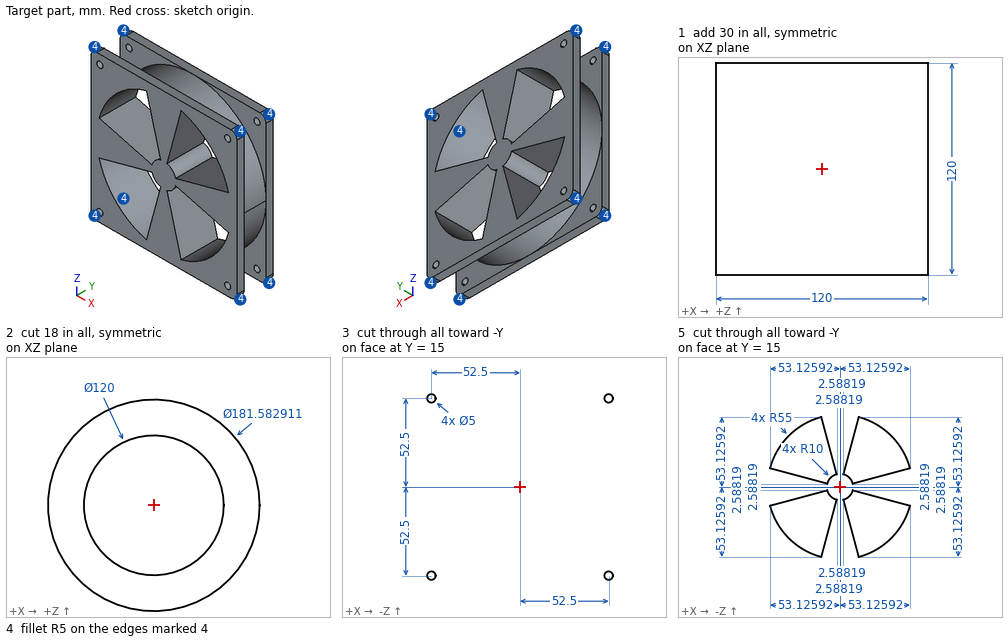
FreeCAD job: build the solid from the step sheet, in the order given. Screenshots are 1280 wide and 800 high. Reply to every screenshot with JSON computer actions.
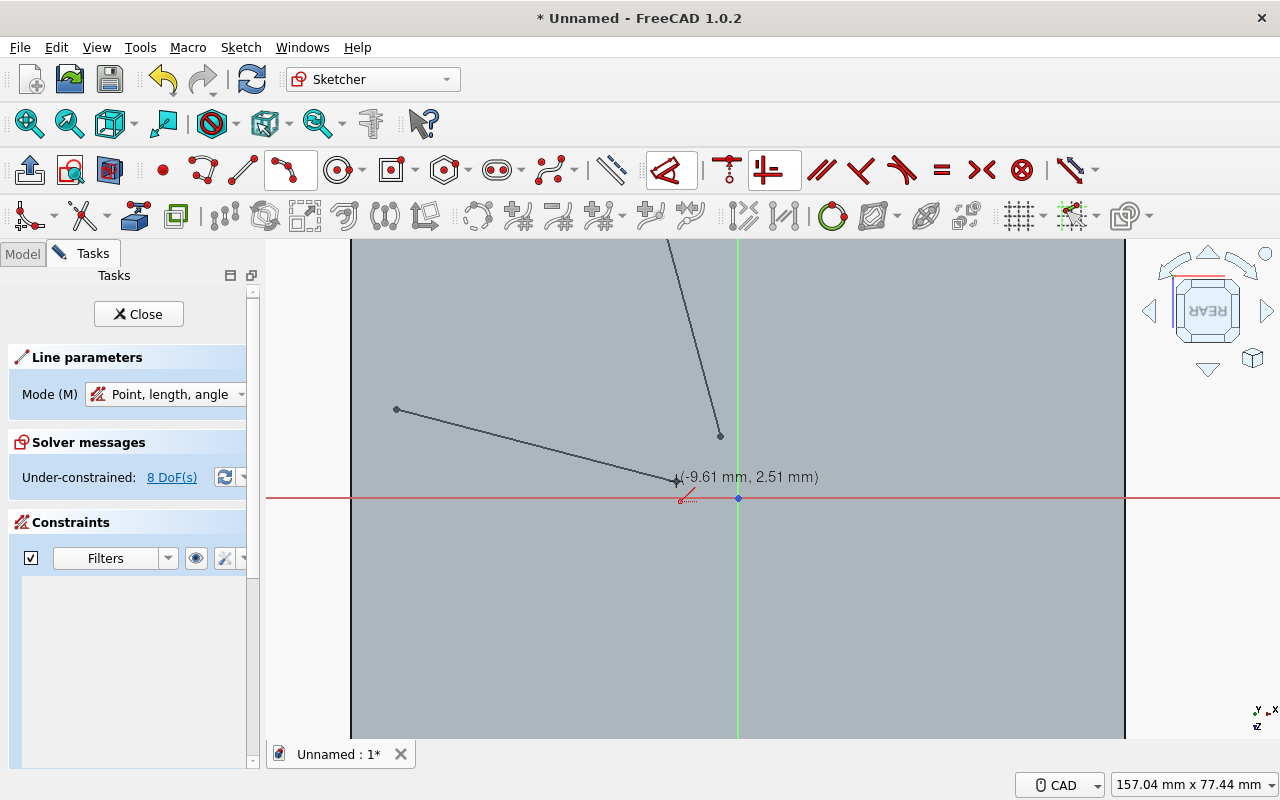
{"action": "left_click", "coordinate": [284, 170]}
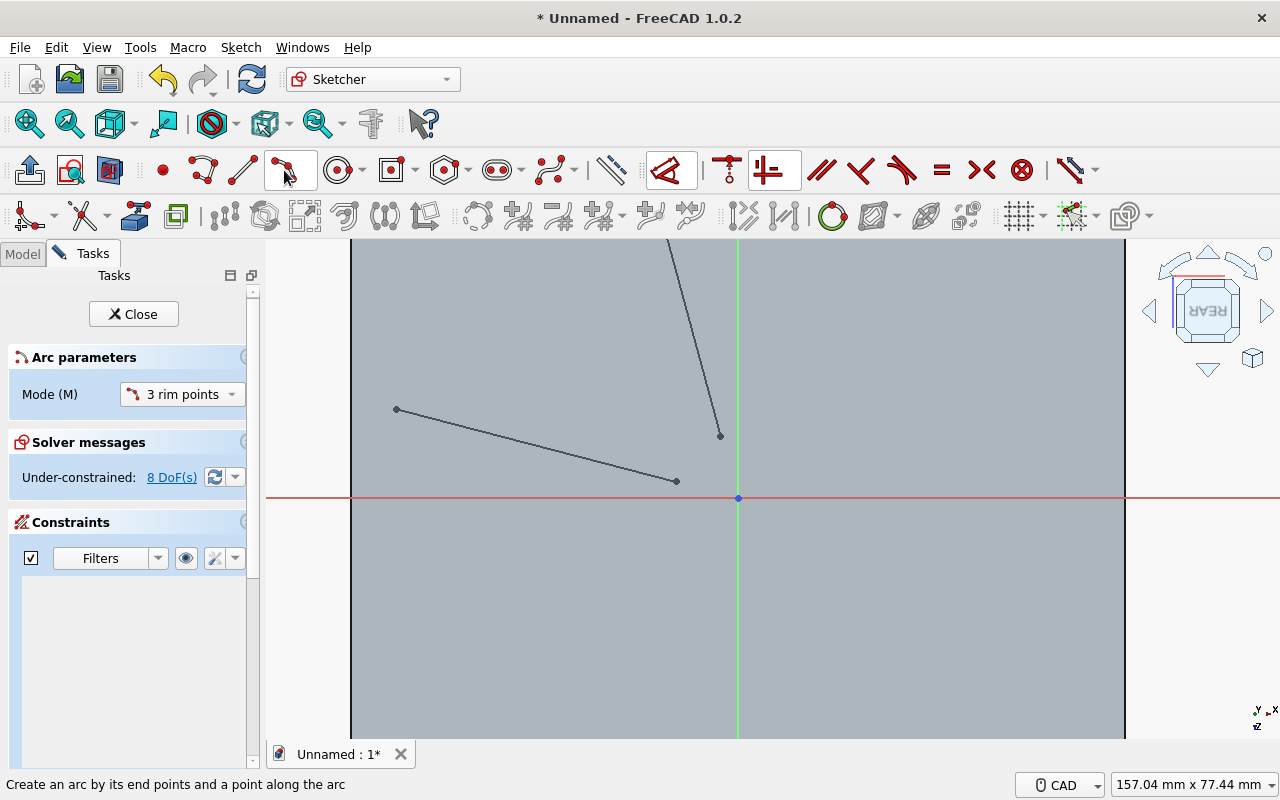
{"action": "scroll", "coordinate": [677, 481], "scroll_direction": "down", "scroll_amount": 4}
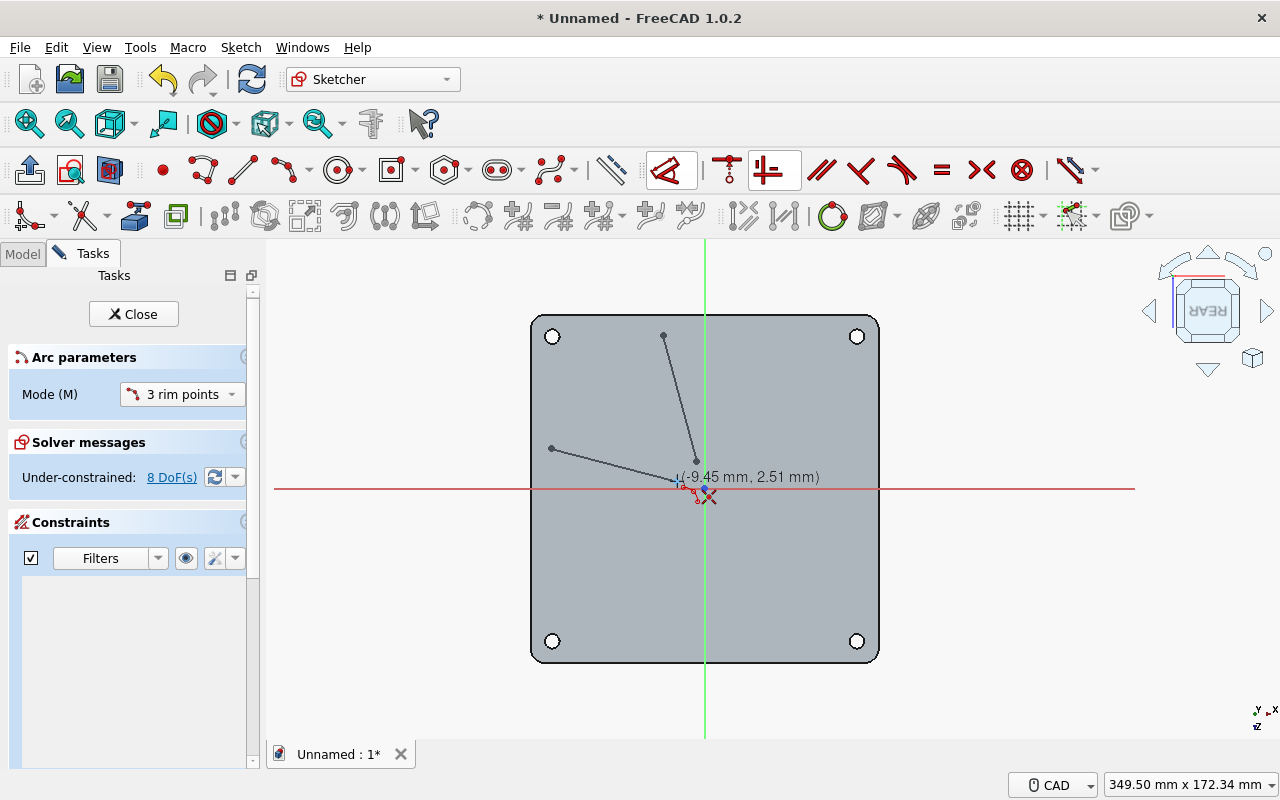
{"action": "left_click", "coordinate": [663, 336]}
{"action": "left_click", "coordinate": [551, 449]}
{"action": "left_click", "coordinate": [592, 376]}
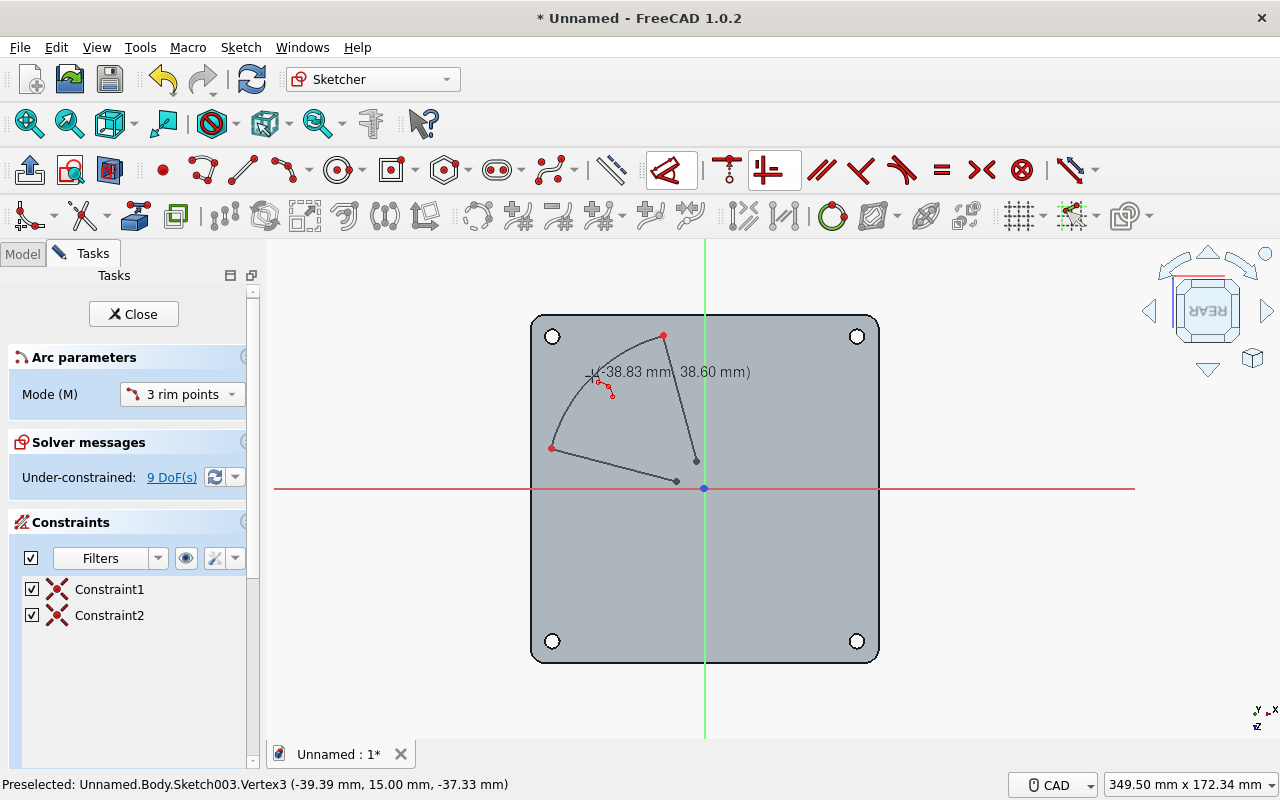
{"action": "scroll", "coordinate": [677, 481], "scroll_direction": "up", "scroll_amount": 4}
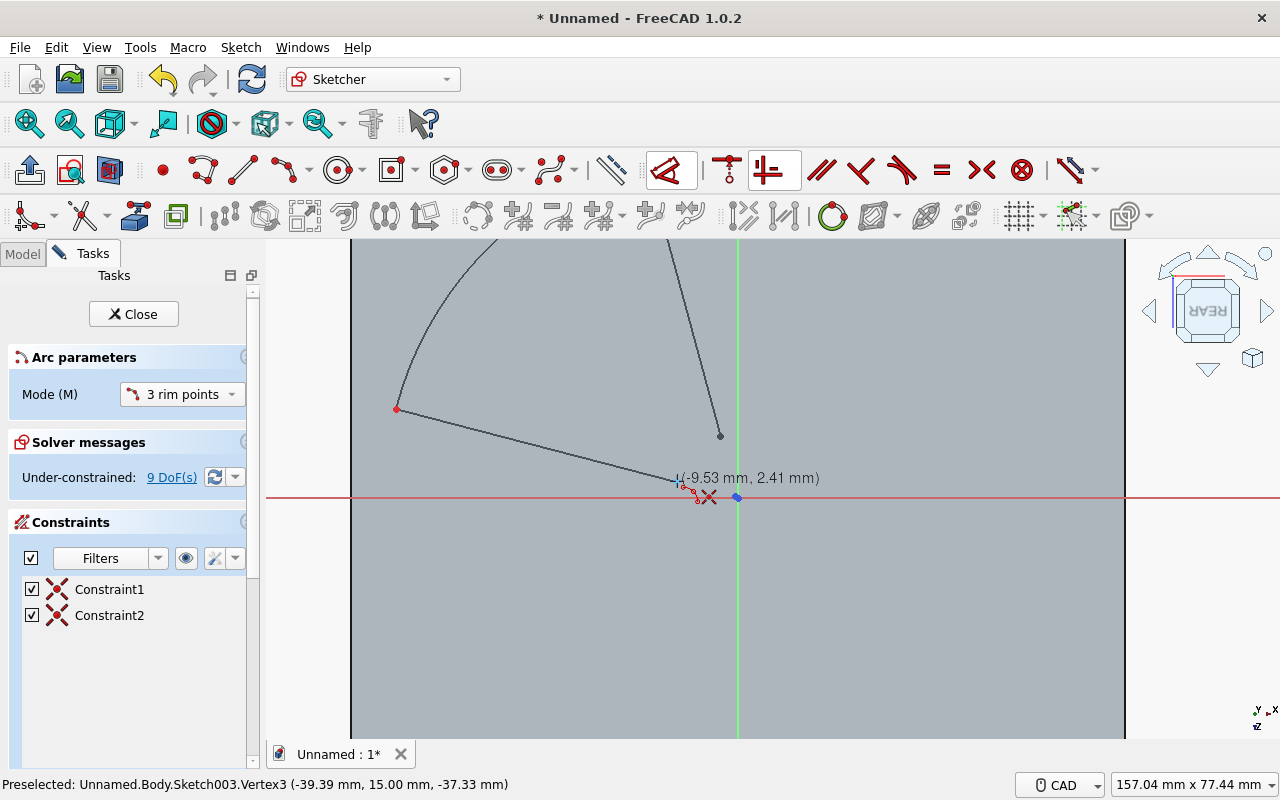
{"action": "left_click", "coordinate": [676, 482]}
{"action": "left_click", "coordinate": [721, 436]}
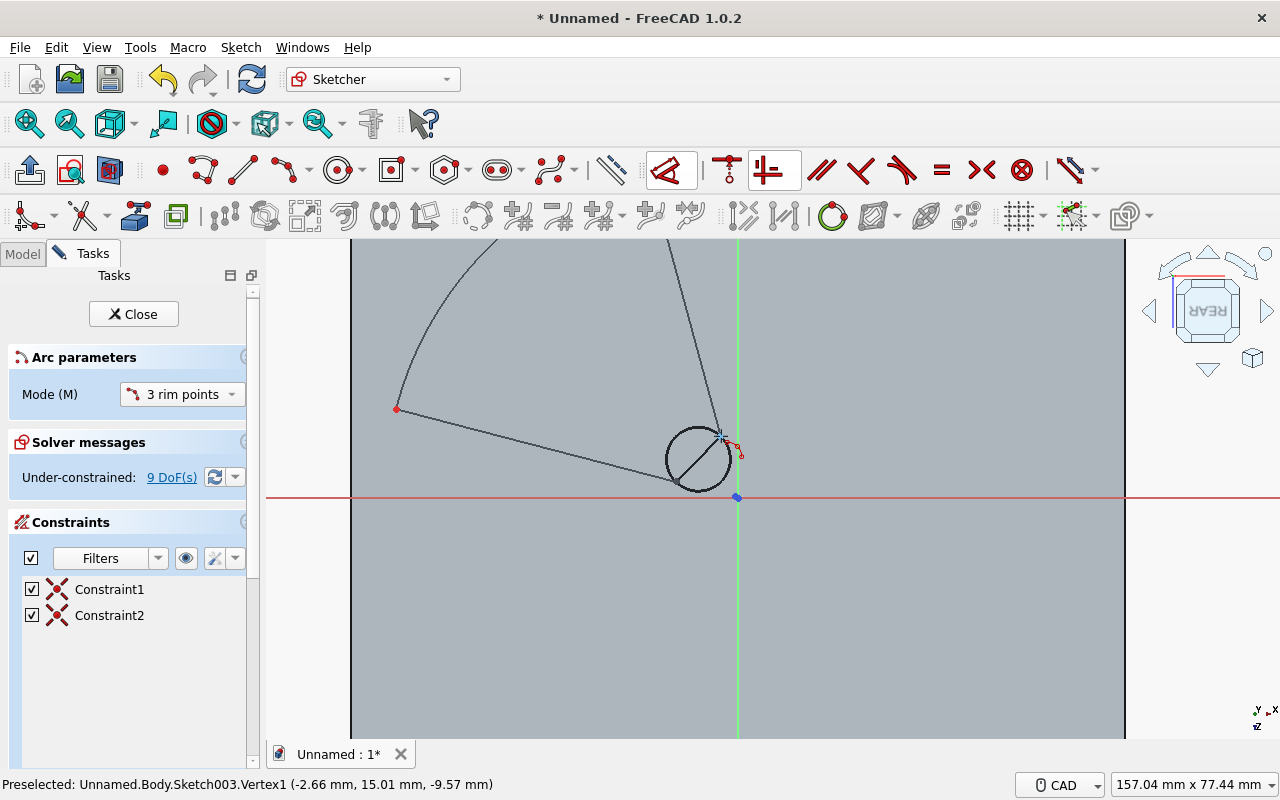
{"action": "scroll", "coordinate": [692, 453], "scroll_direction": "up", "scroll_amount": 4}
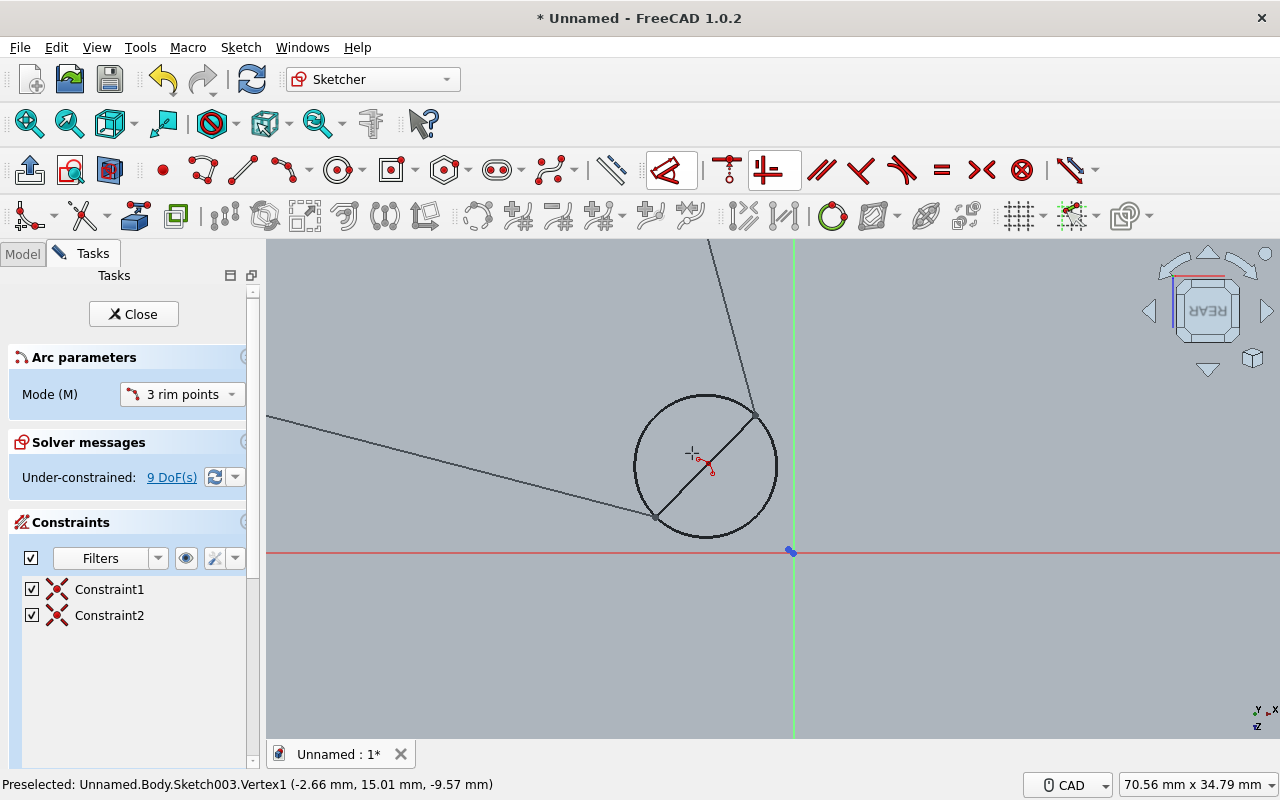
{"action": "left_click", "coordinate": [692, 451]}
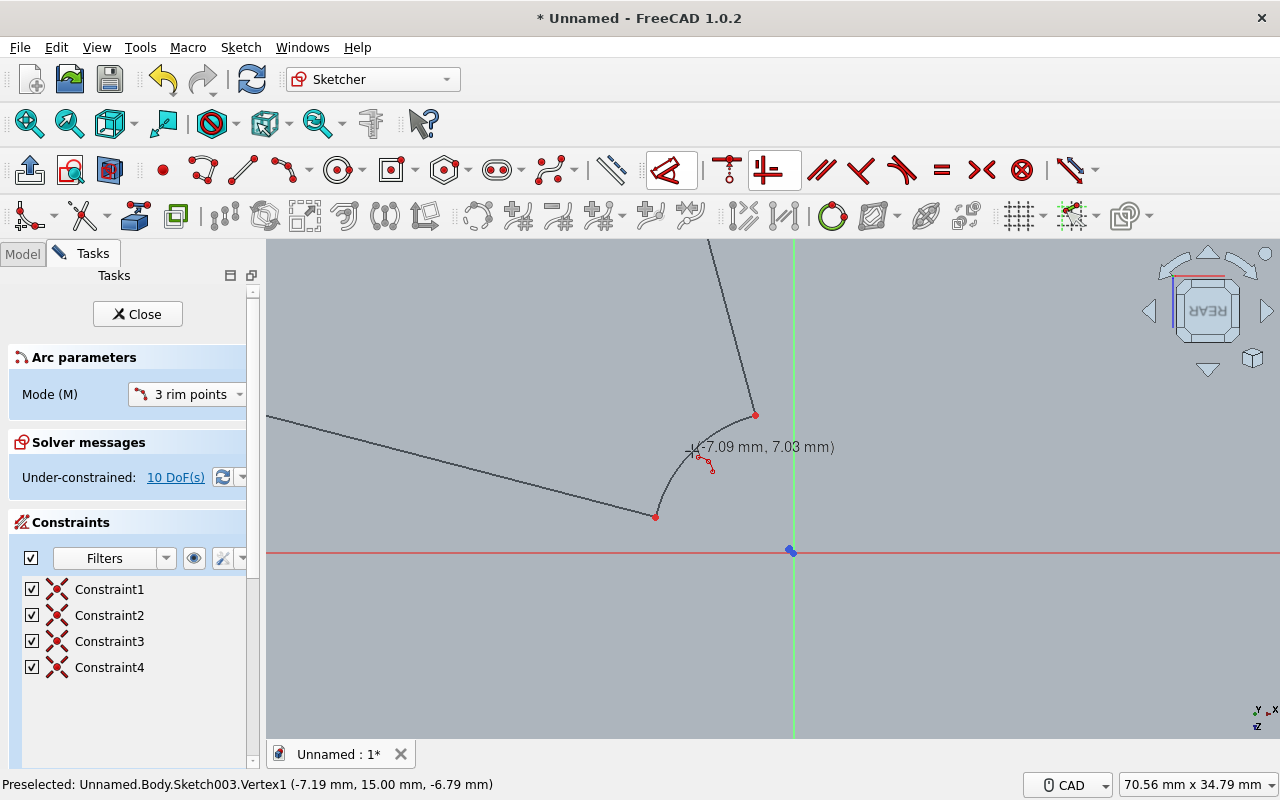
{"action": "left_click", "coordinate": [244, 170]}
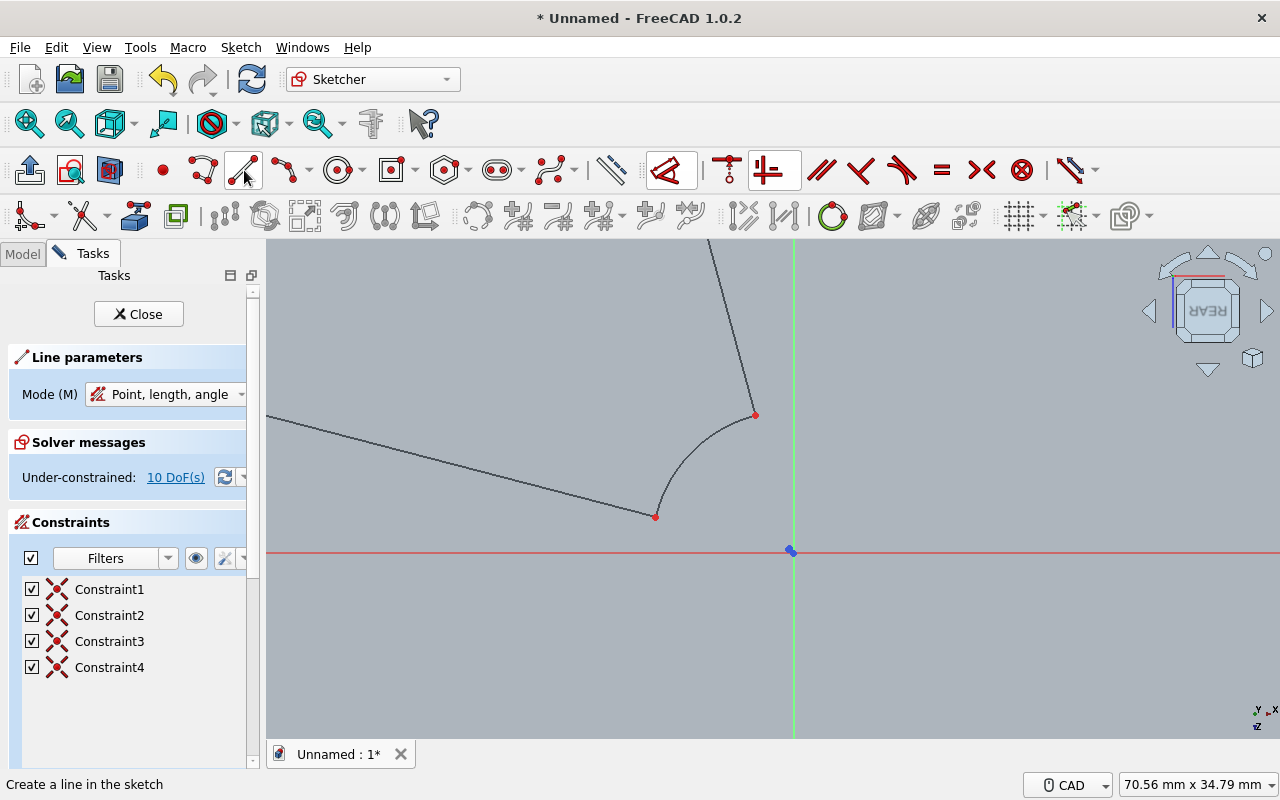
{"action": "scroll", "coordinate": [682, 473], "scroll_direction": "down", "scroll_amount": 8}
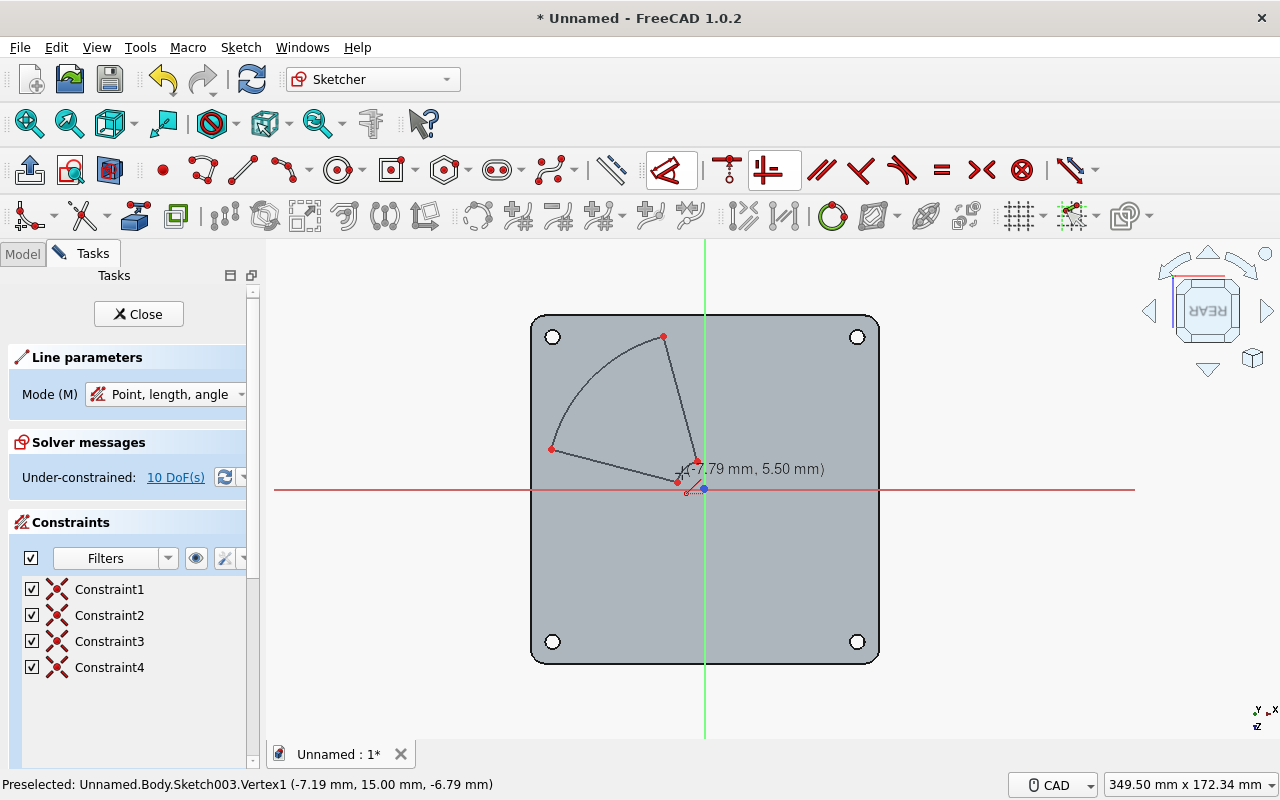
{"action": "left_click", "coordinate": [746, 335]}